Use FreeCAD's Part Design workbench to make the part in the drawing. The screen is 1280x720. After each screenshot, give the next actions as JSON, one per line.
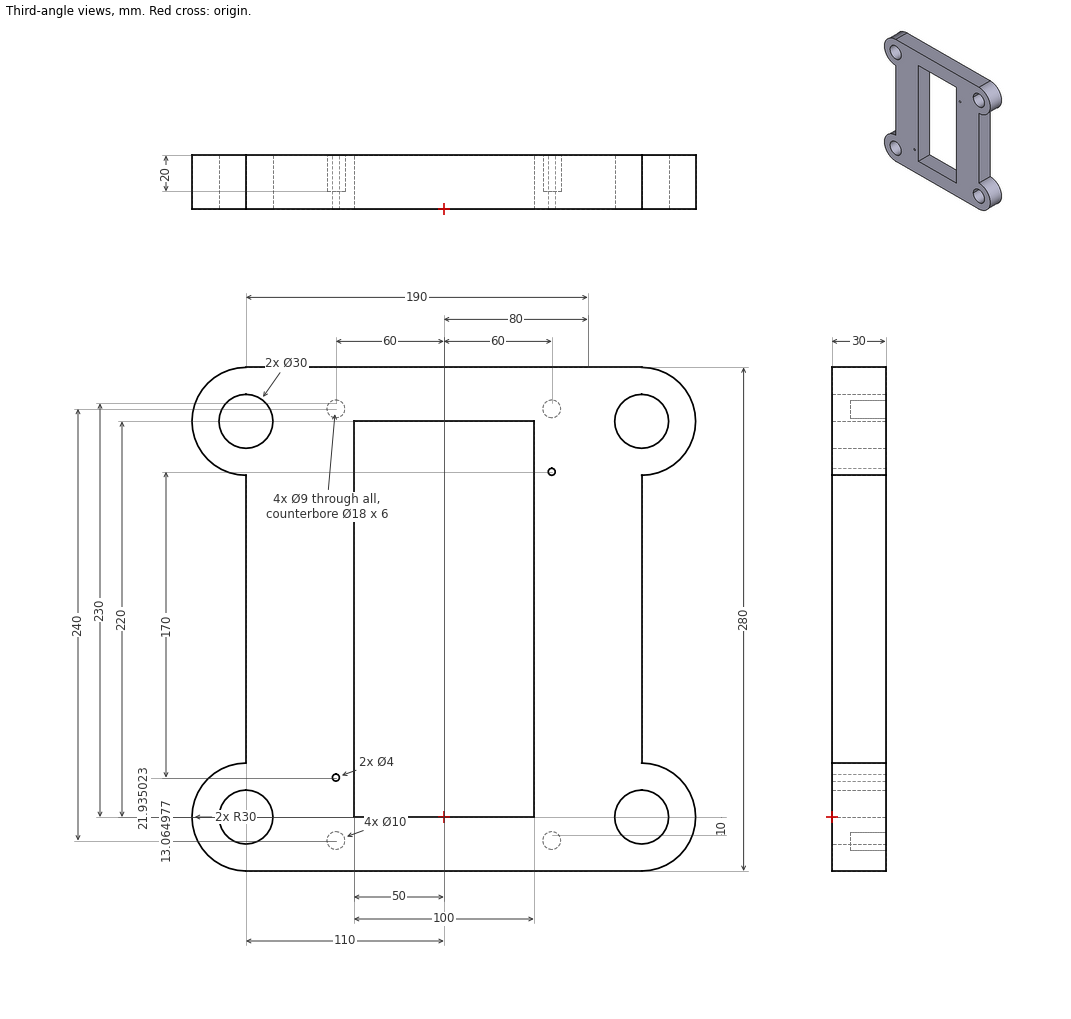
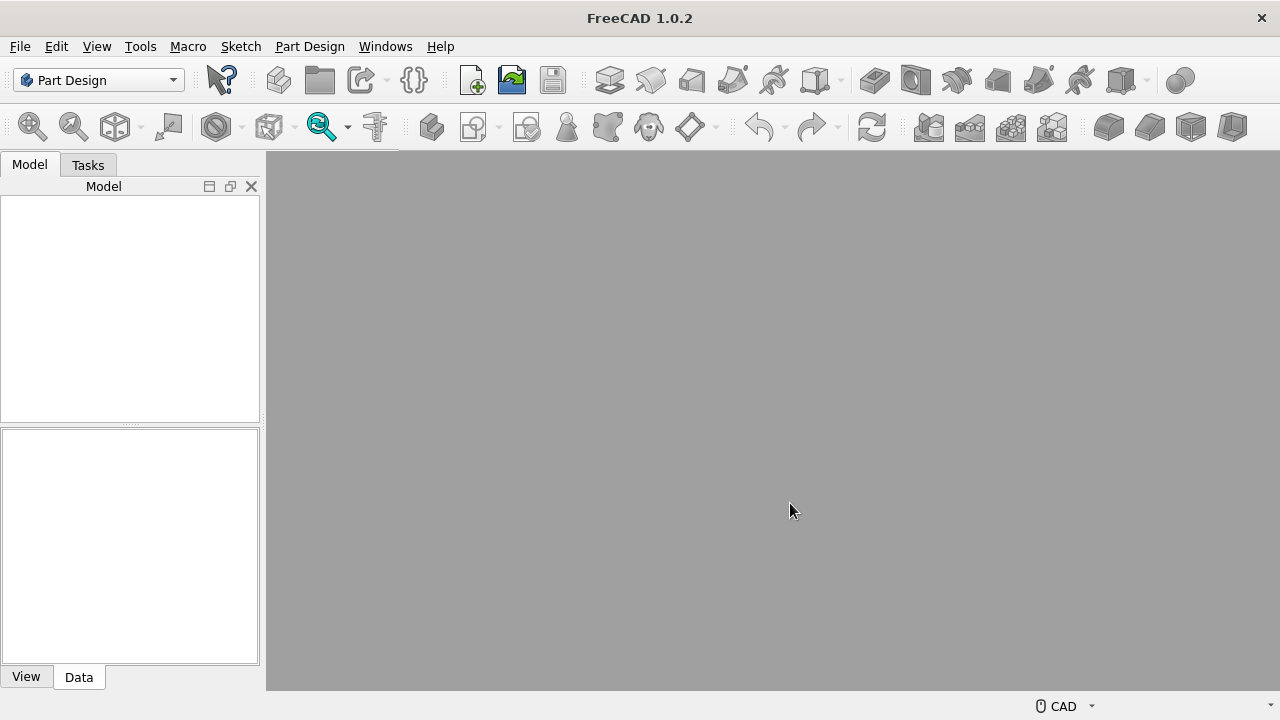
{"action": "left_click", "coordinate": [471, 80]}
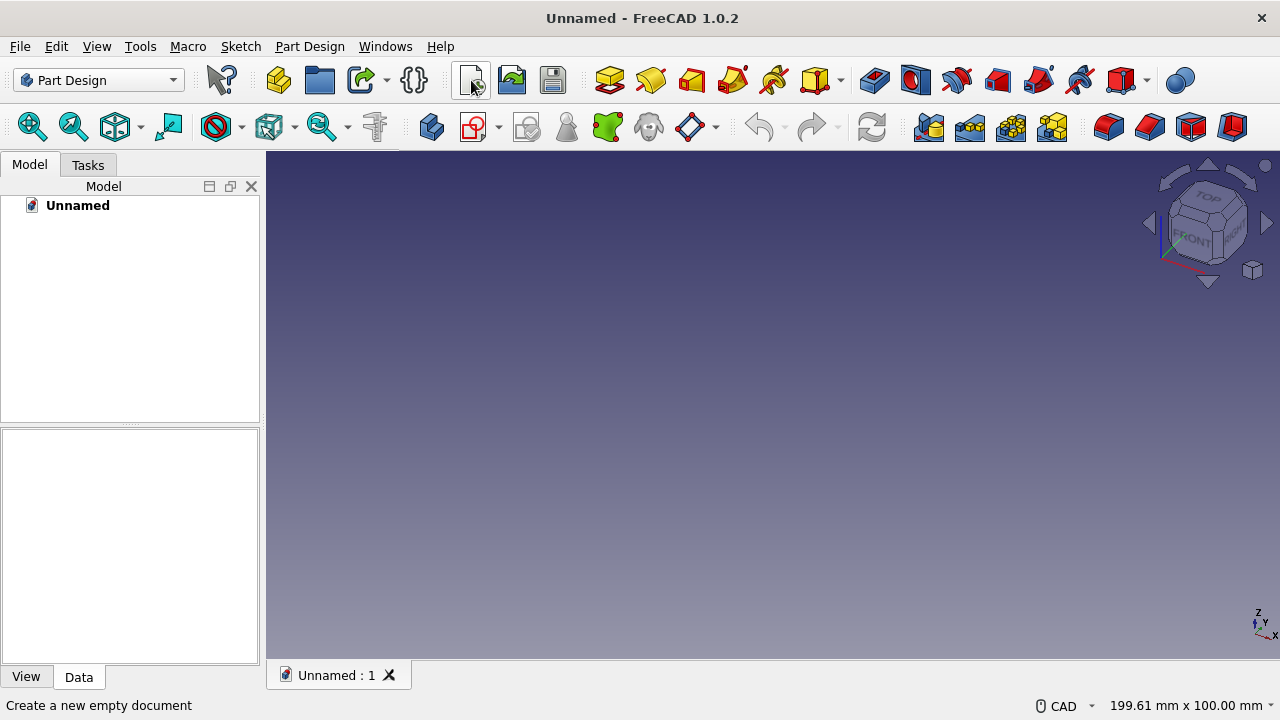
{"action": "left_click", "coordinate": [472, 128]}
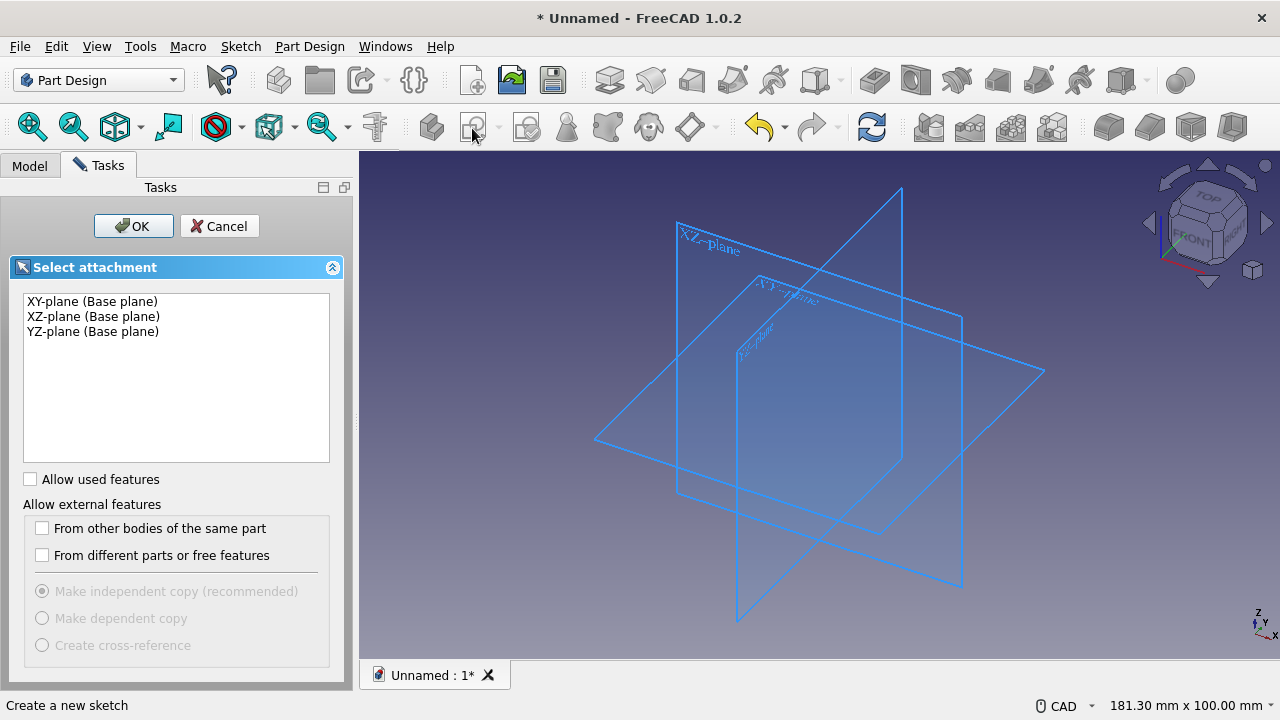
{"action": "left_click", "coordinate": [84, 316]}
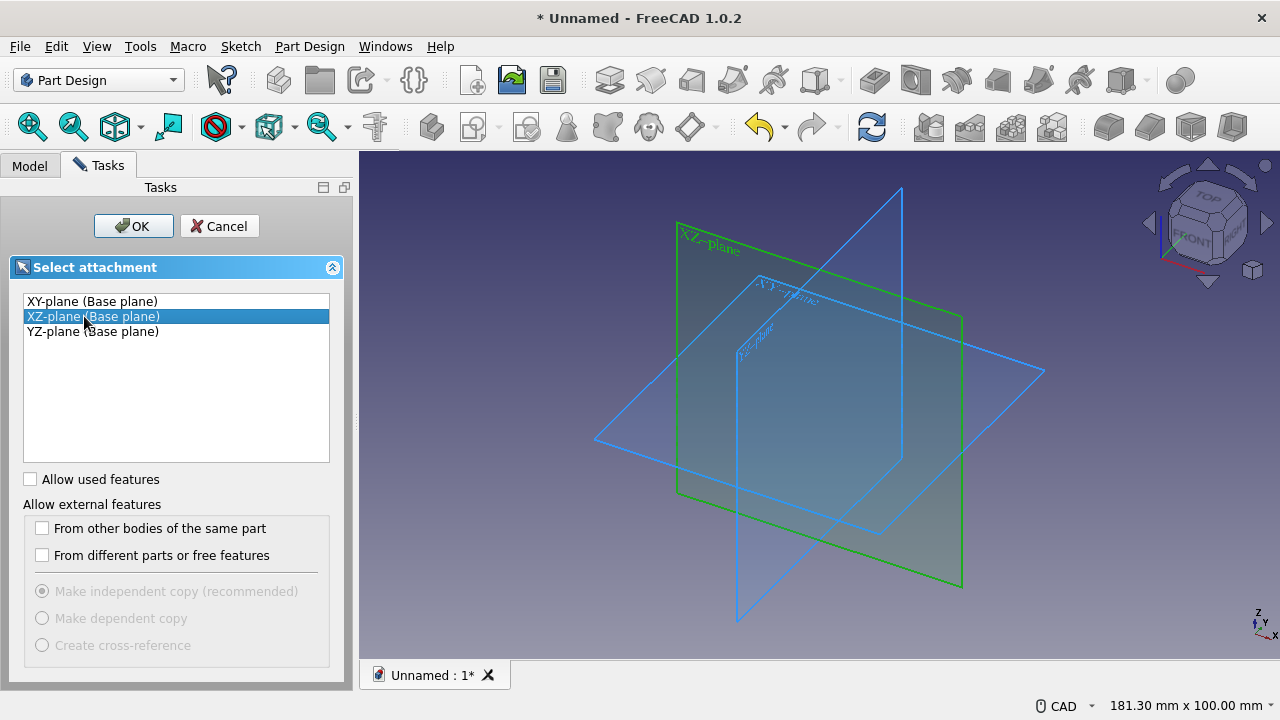
{"action": "left_click", "coordinate": [134, 226]}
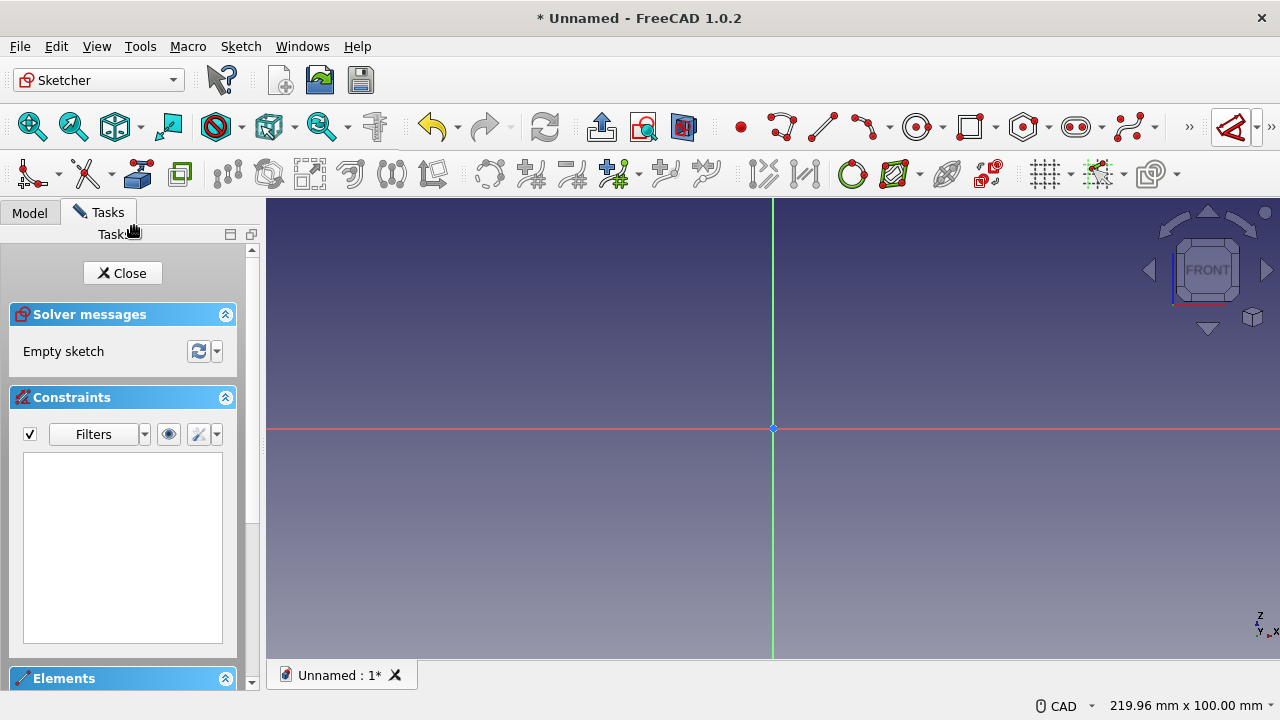
{"action": "scroll", "coordinate": [722, 557], "scroll_direction": "down", "scroll_amount": 8}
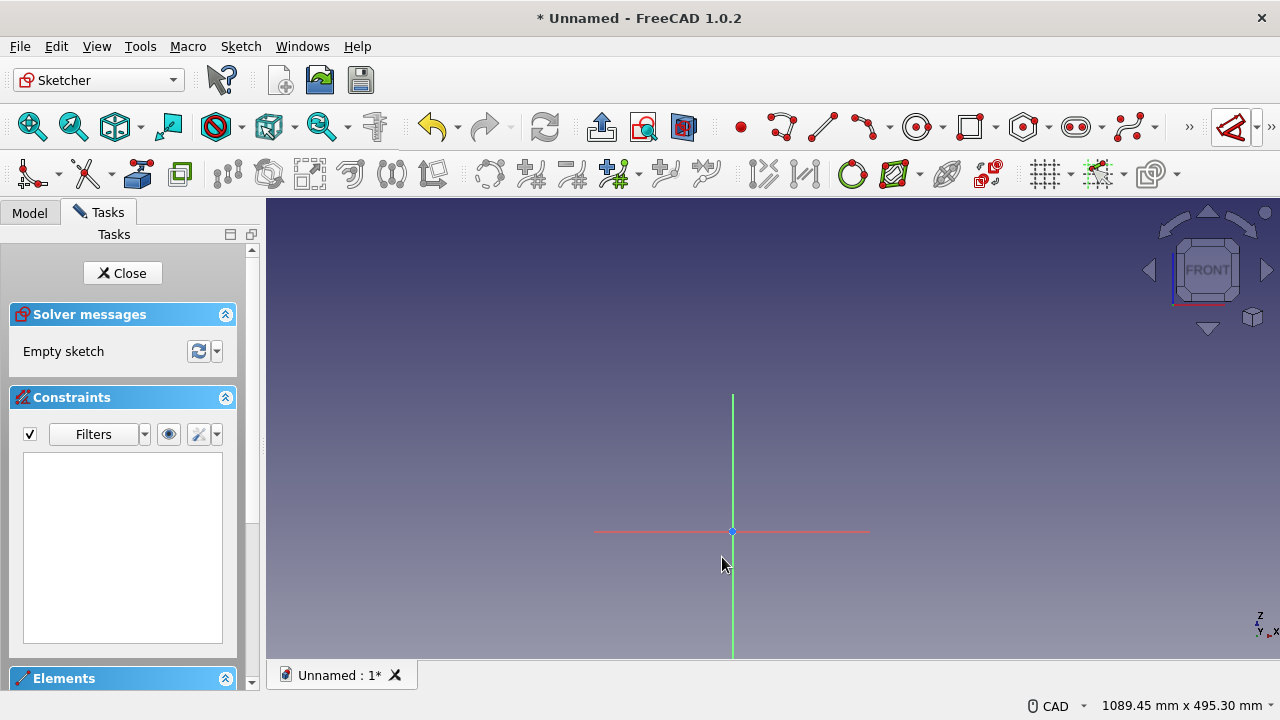
{"action": "key", "text": "g m"}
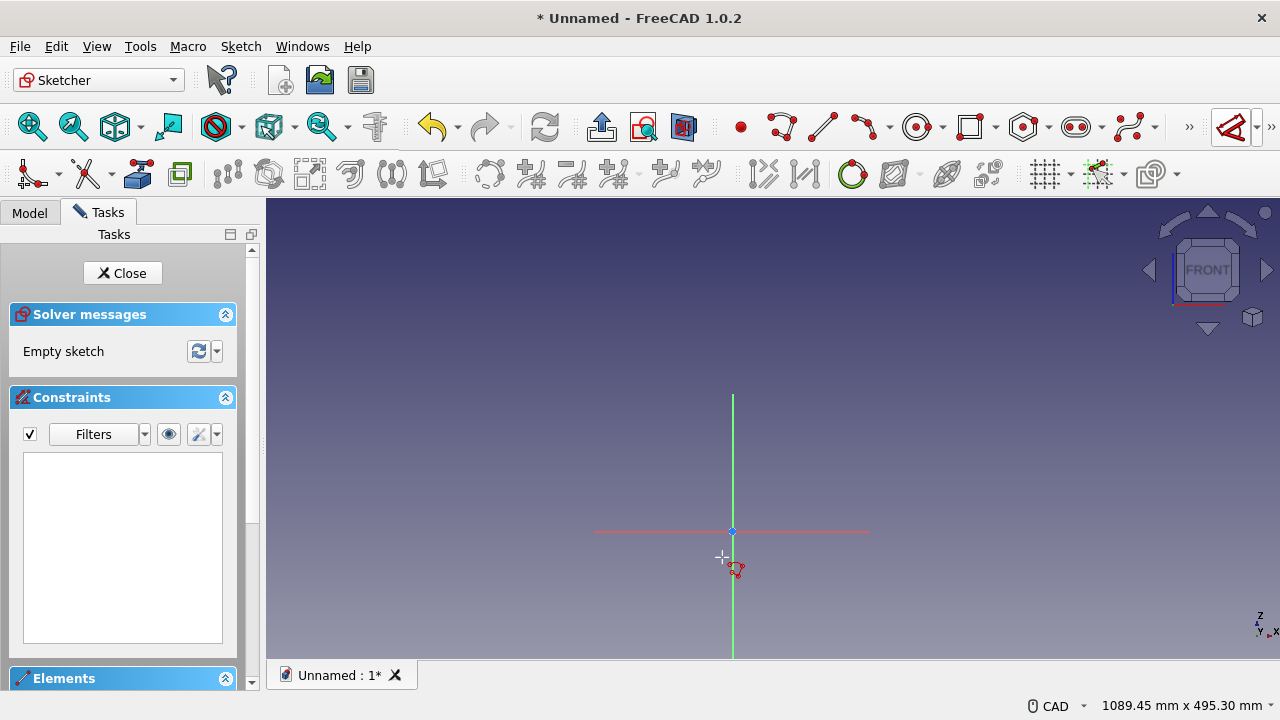
{"action": "left_click", "coordinate": [630, 299]}
{"action": "left_click", "coordinate": [807, 299]}
{"action": "left_click", "coordinate": [807, 560]}
{"action": "left_click", "coordinate": [630, 560]}
{"action": "right_click", "coordinate": [630, 560]}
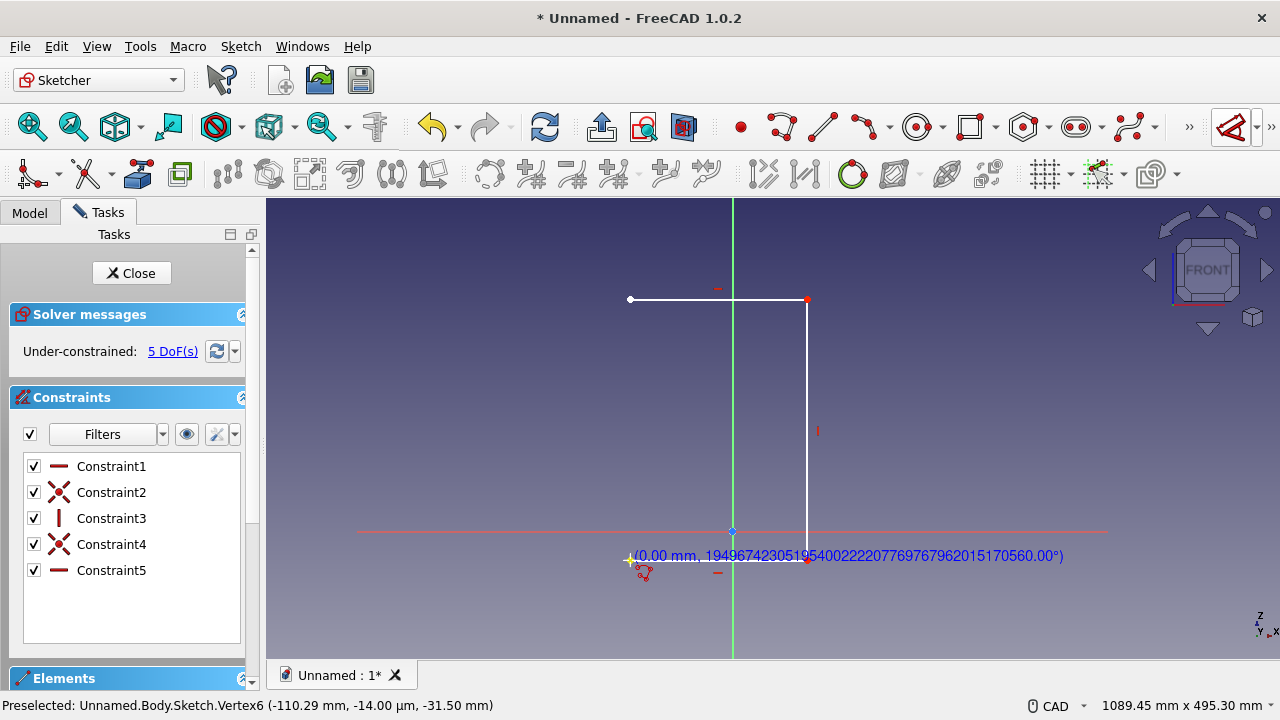
{"action": "key", "text": "g l"}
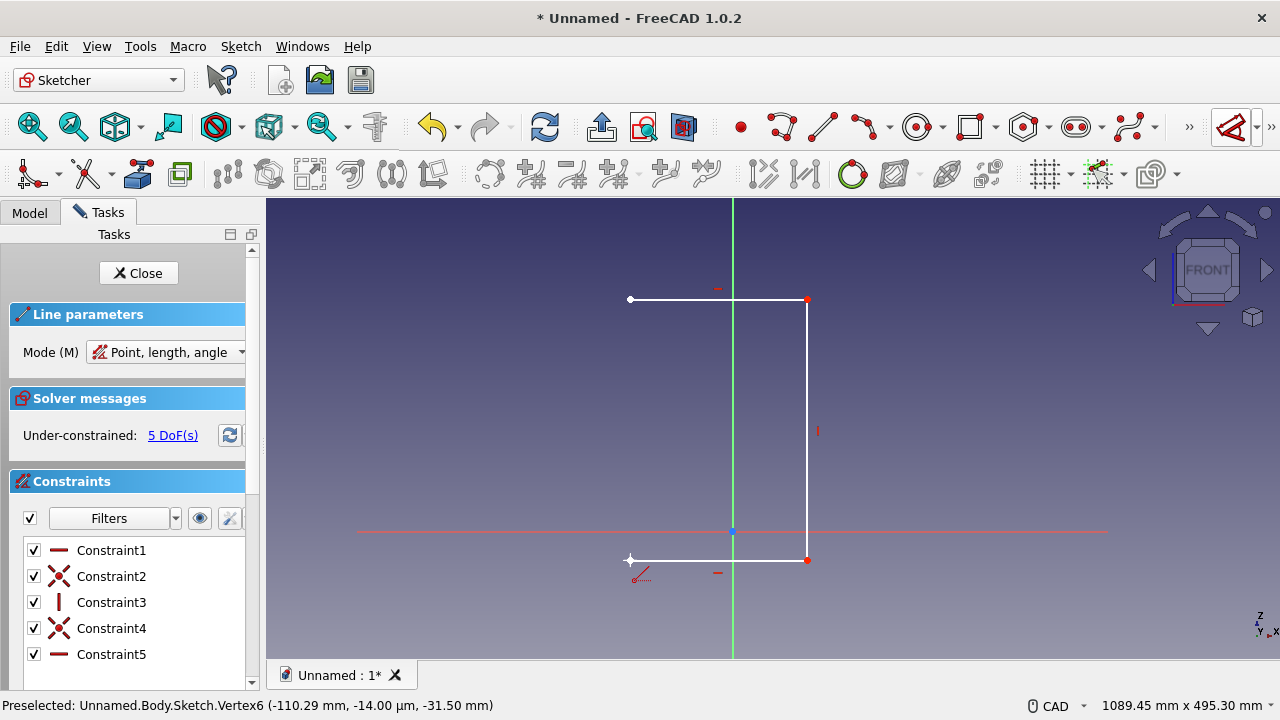
{"action": "left_click", "coordinate": [630, 504]}
{"action": "left_click", "coordinate": [630, 355]}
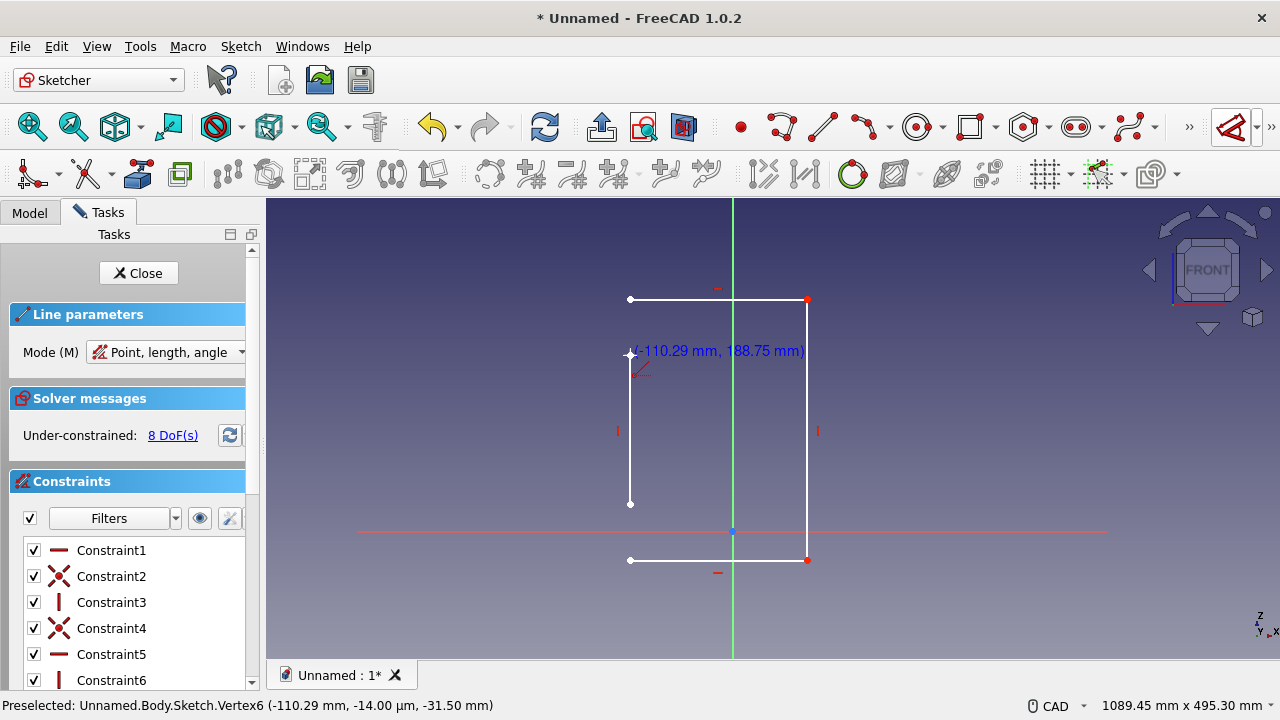
{"action": "key", "text": "g 3 a"}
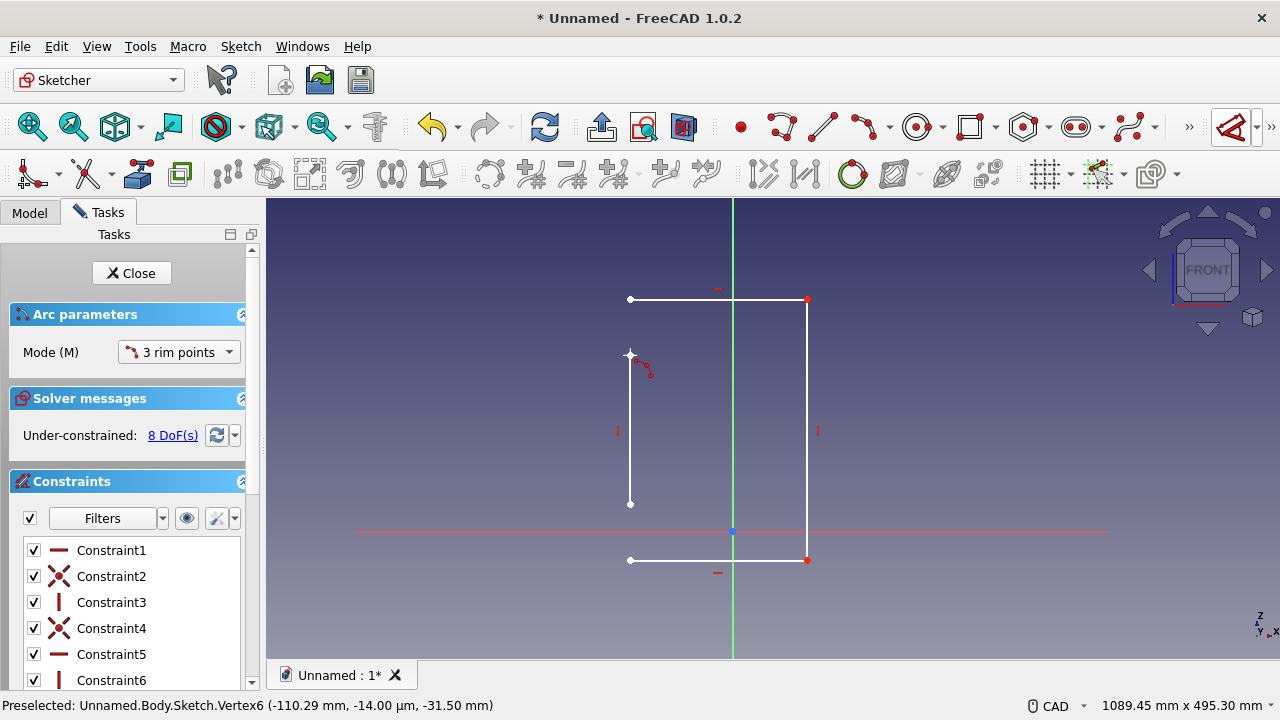
{"action": "left_click", "coordinate": [630, 561]}
{"action": "left_click", "coordinate": [630, 505]}
{"action": "left_click", "coordinate": [608, 515]}